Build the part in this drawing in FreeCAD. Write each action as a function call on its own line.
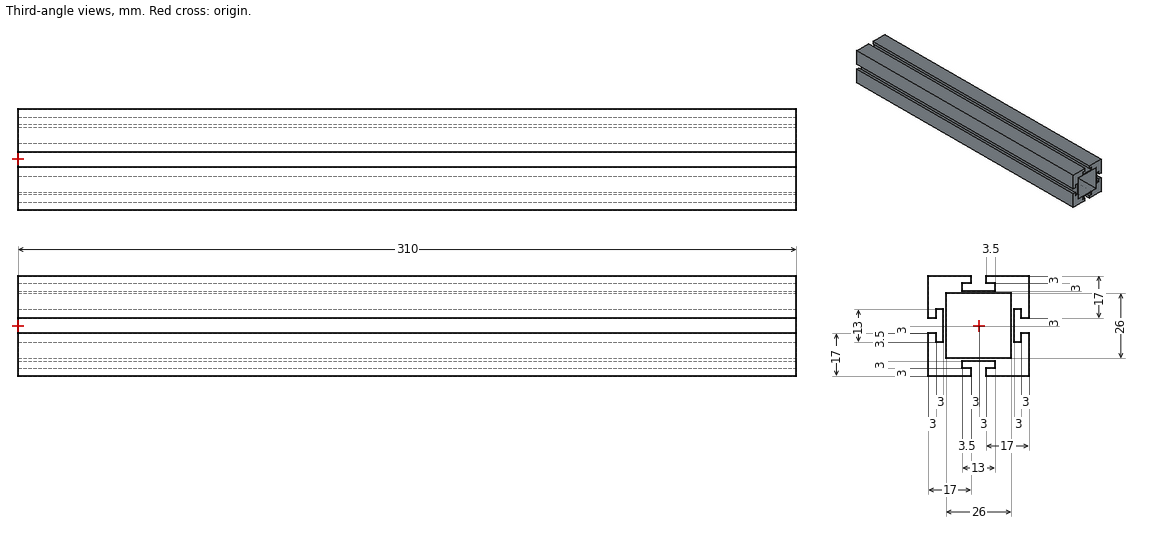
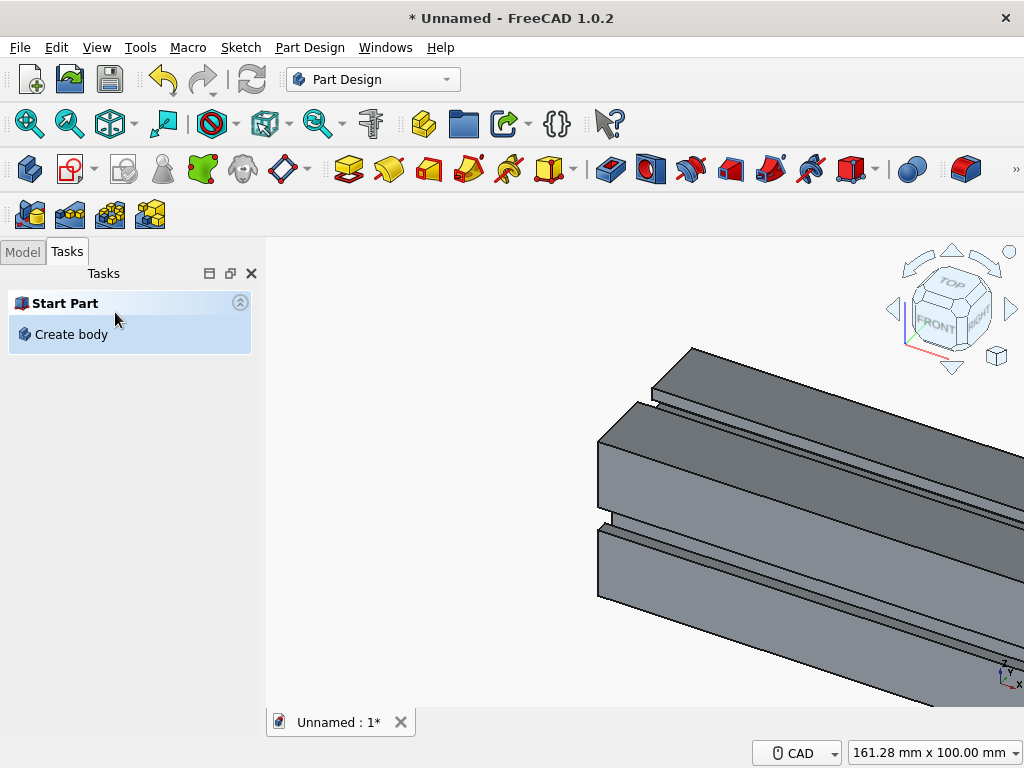
key(0)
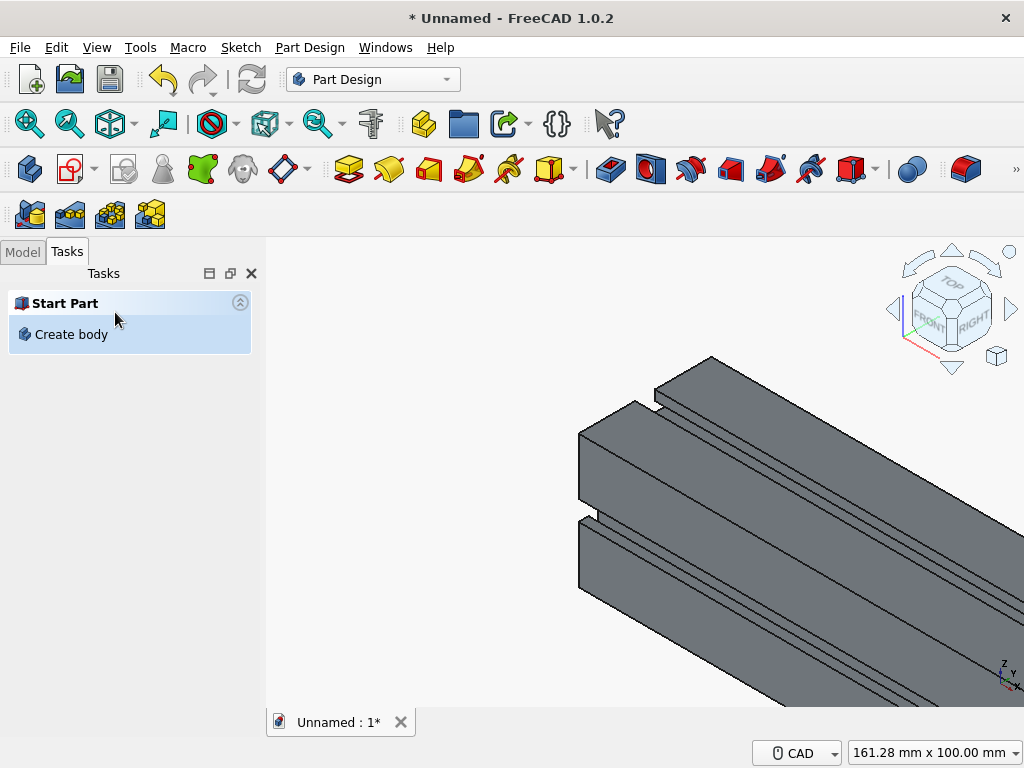
click(30, 124)